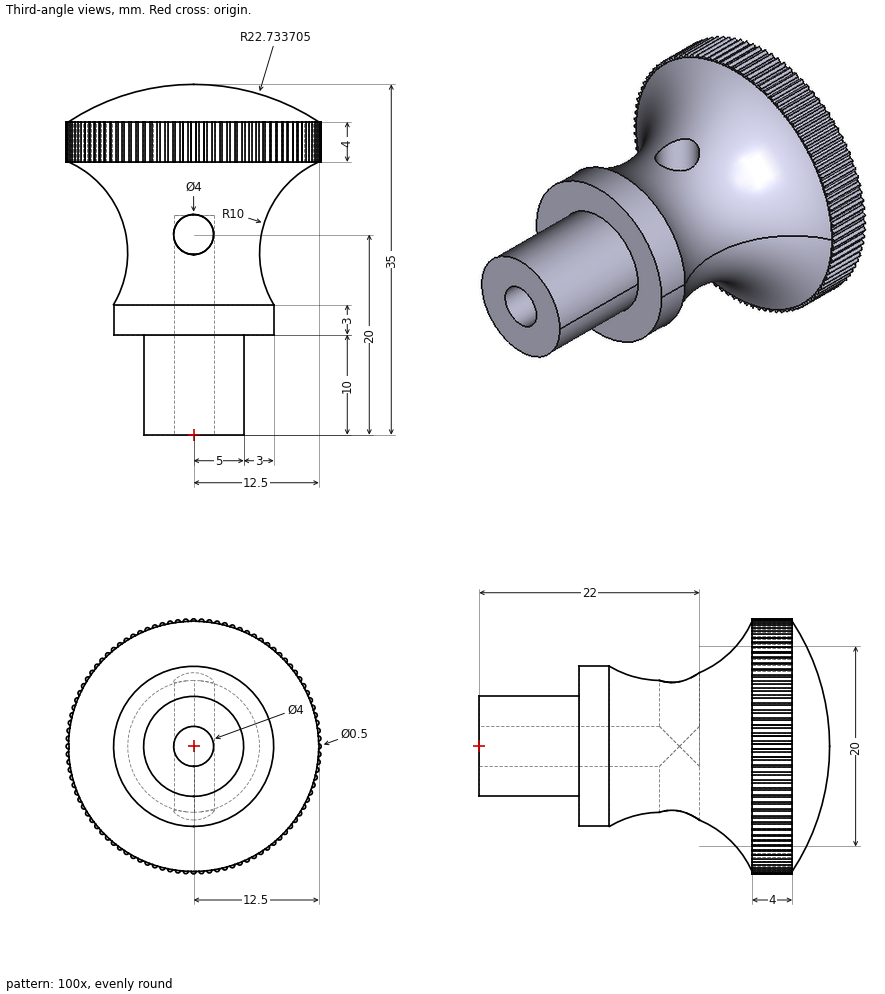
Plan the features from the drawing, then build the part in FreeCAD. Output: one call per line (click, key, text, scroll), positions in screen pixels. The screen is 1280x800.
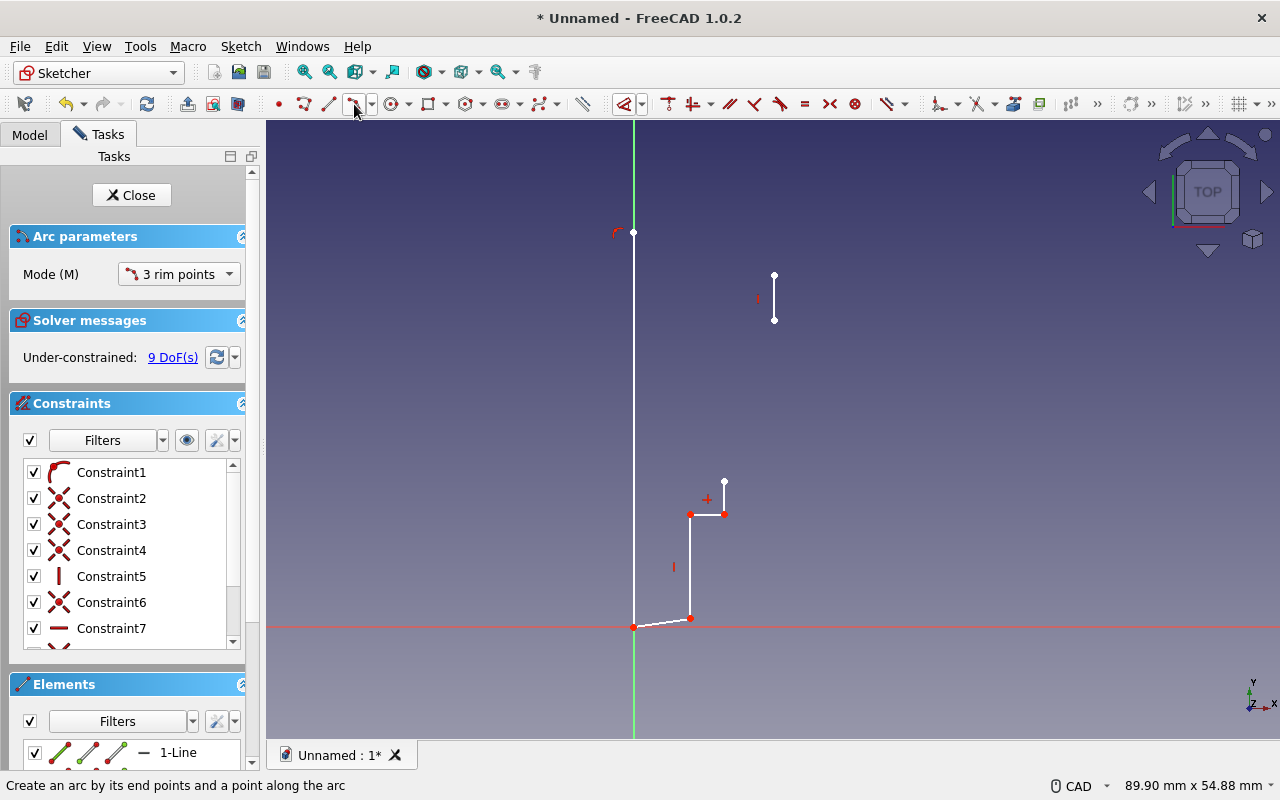
click(724, 482)
click(774, 321)
click(713, 389)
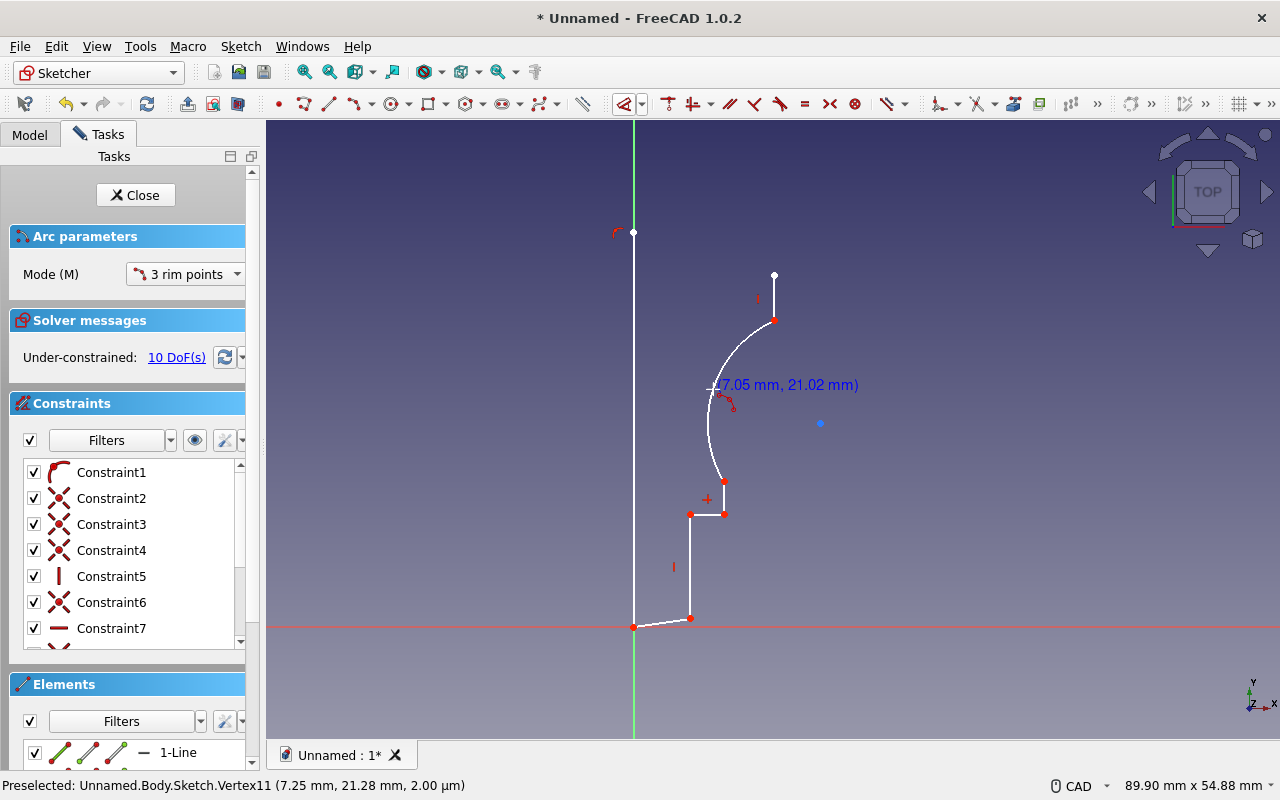
click(774, 276)
click(634, 233)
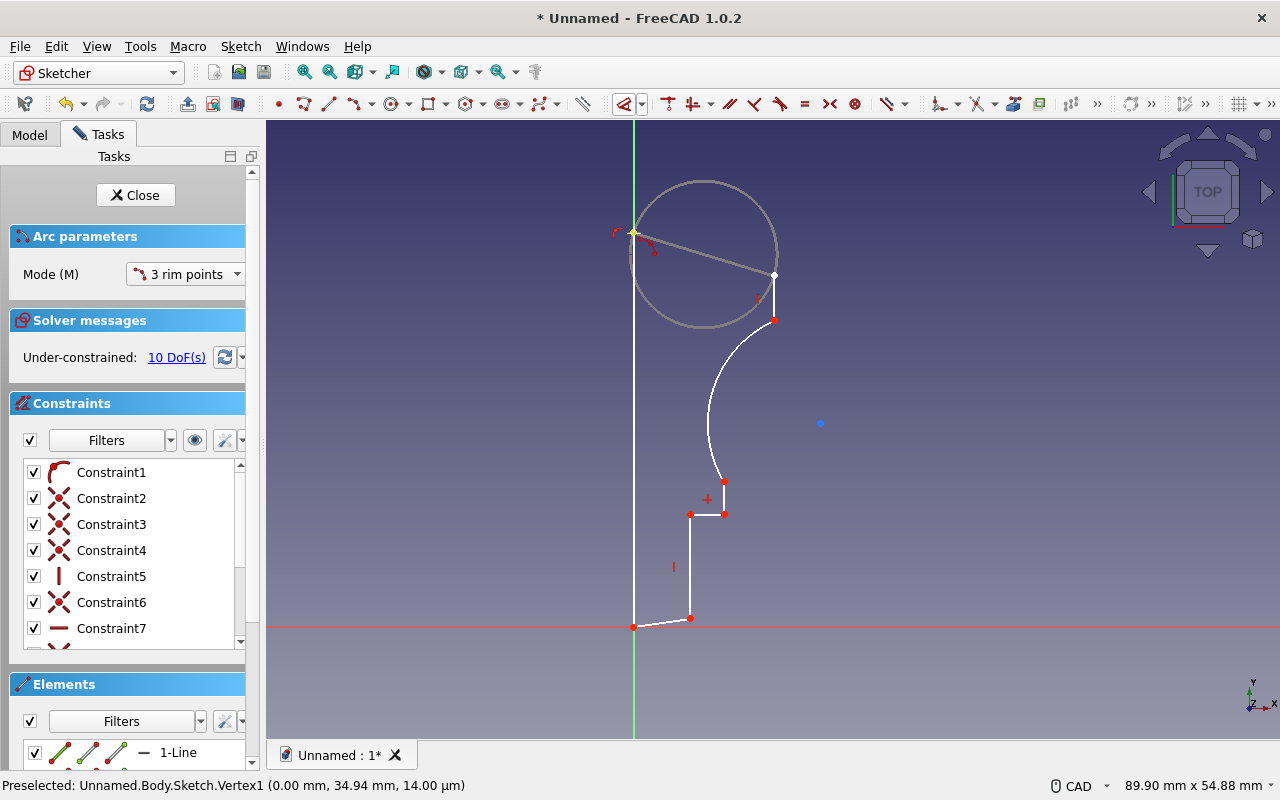
scroll(707, 243, up, 2)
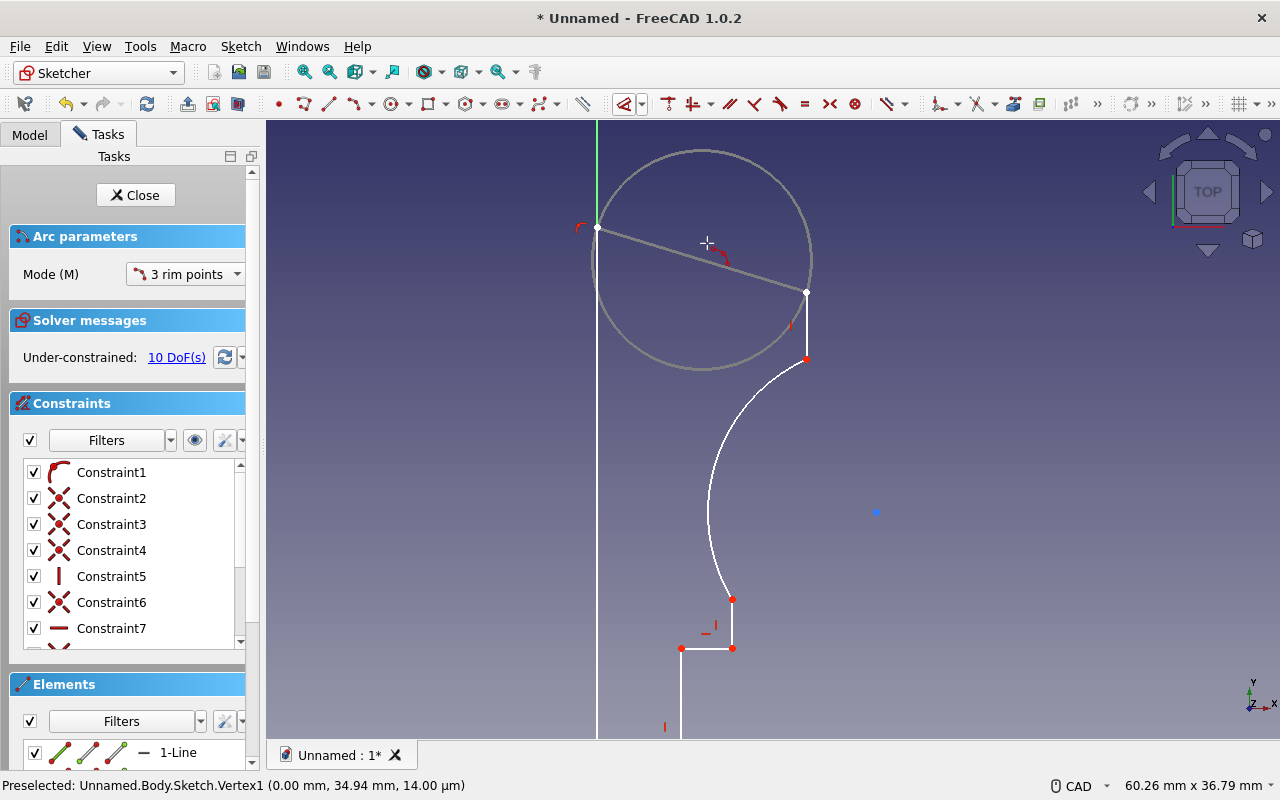
click(707, 243)
key(Escape)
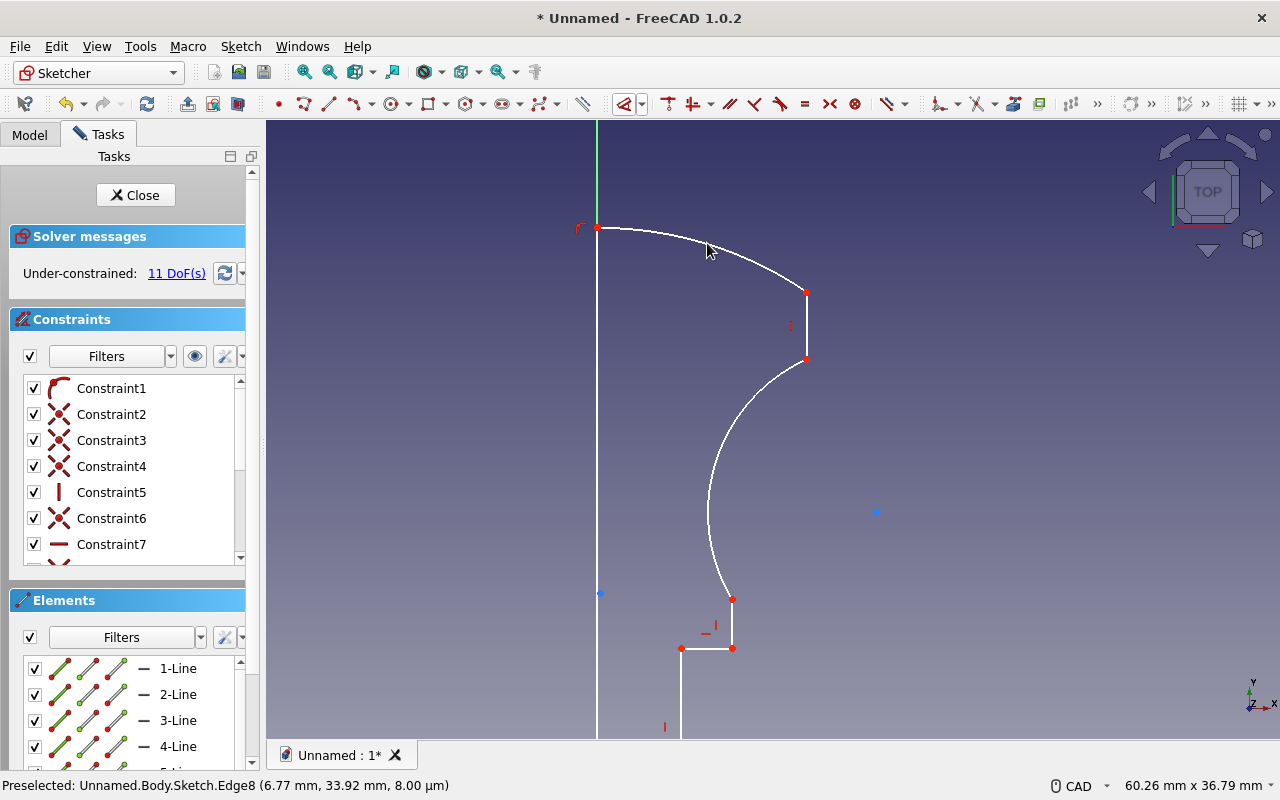
scroll(709, 242, down, 2)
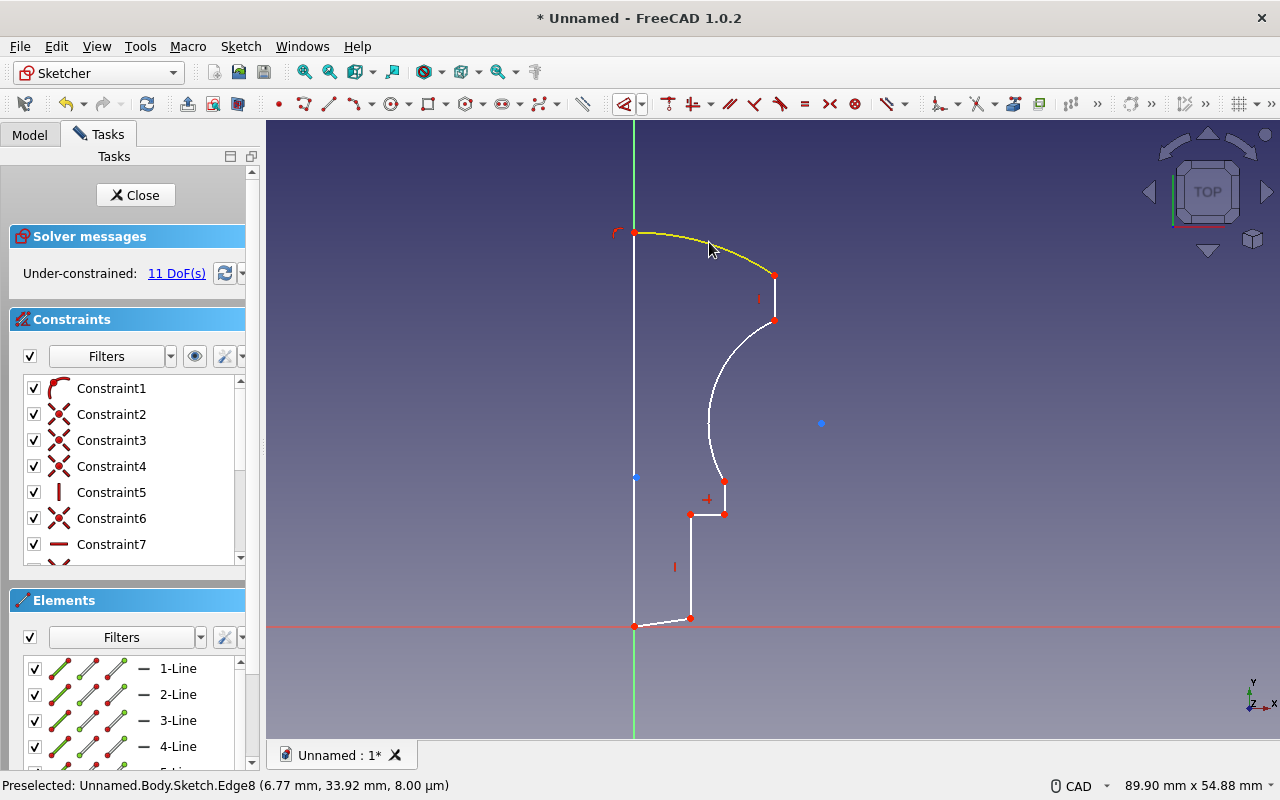
click(651, 624)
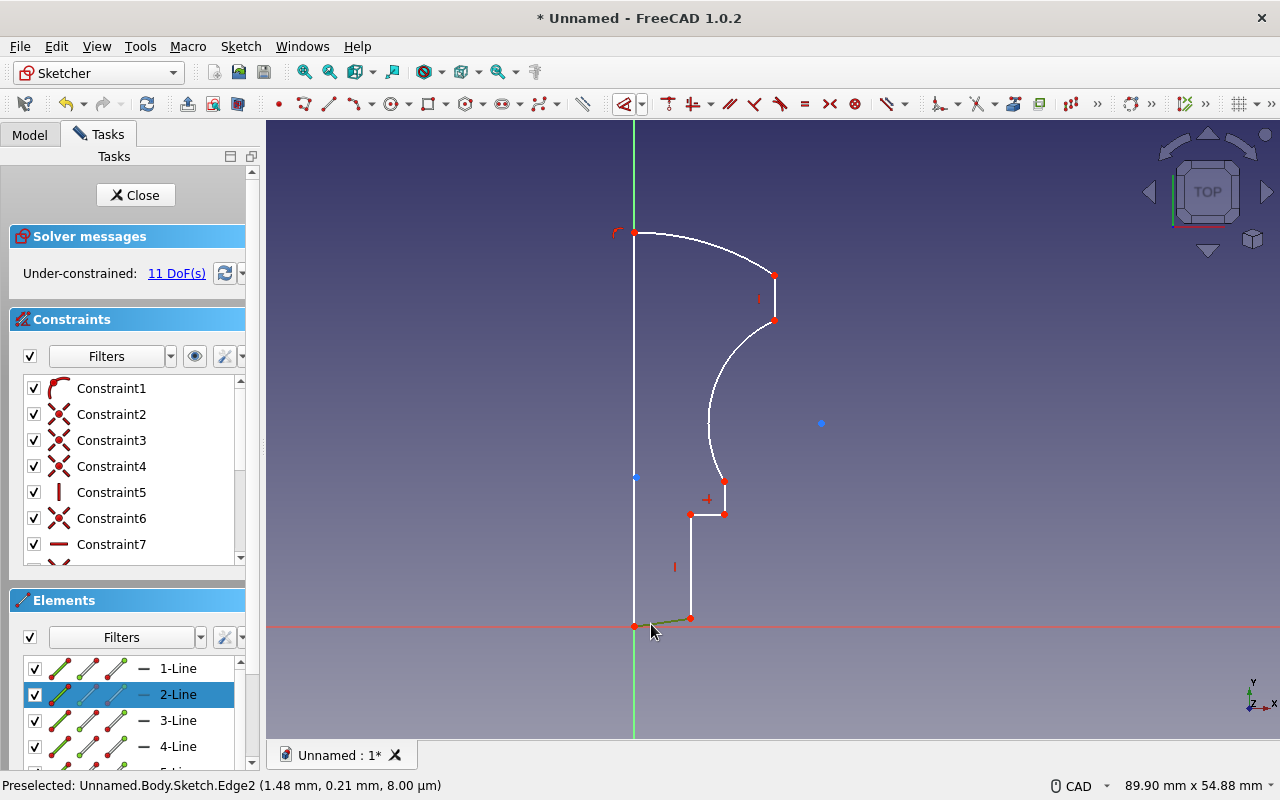
key(h)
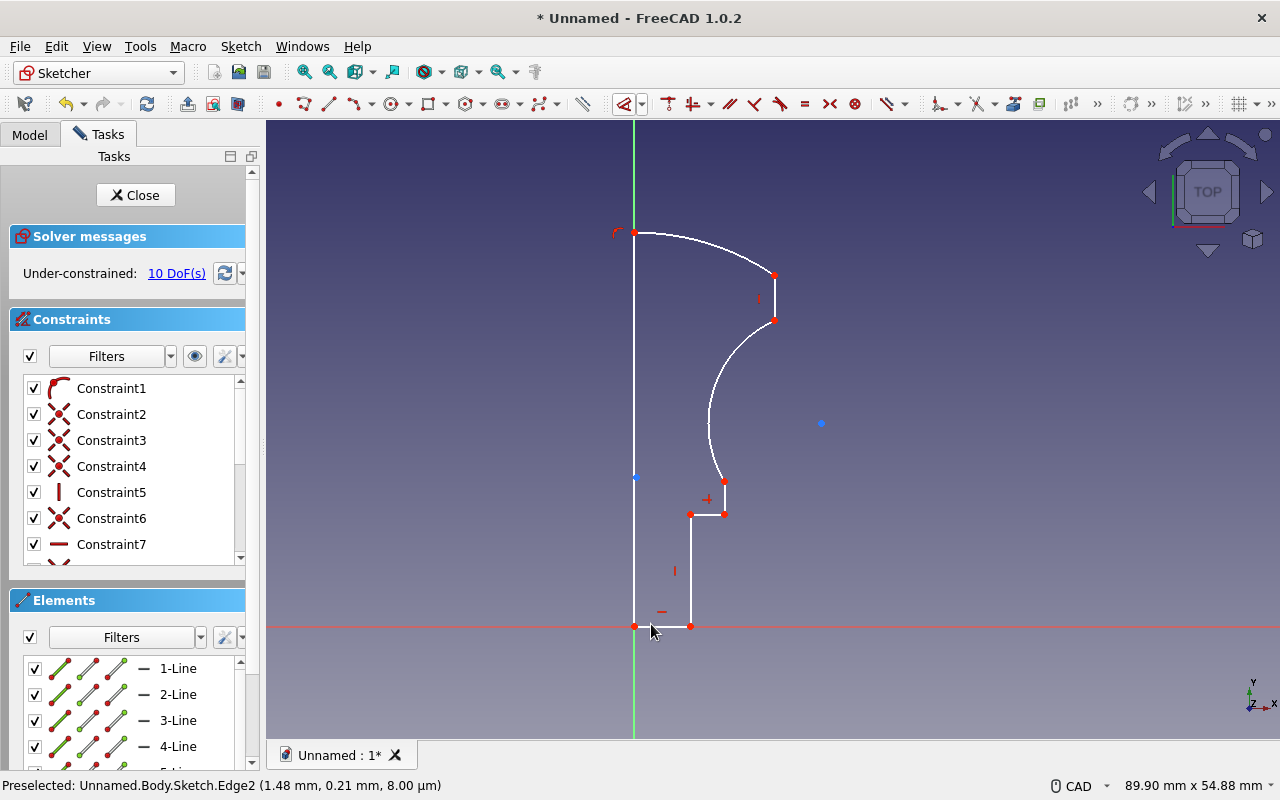
click(636, 477)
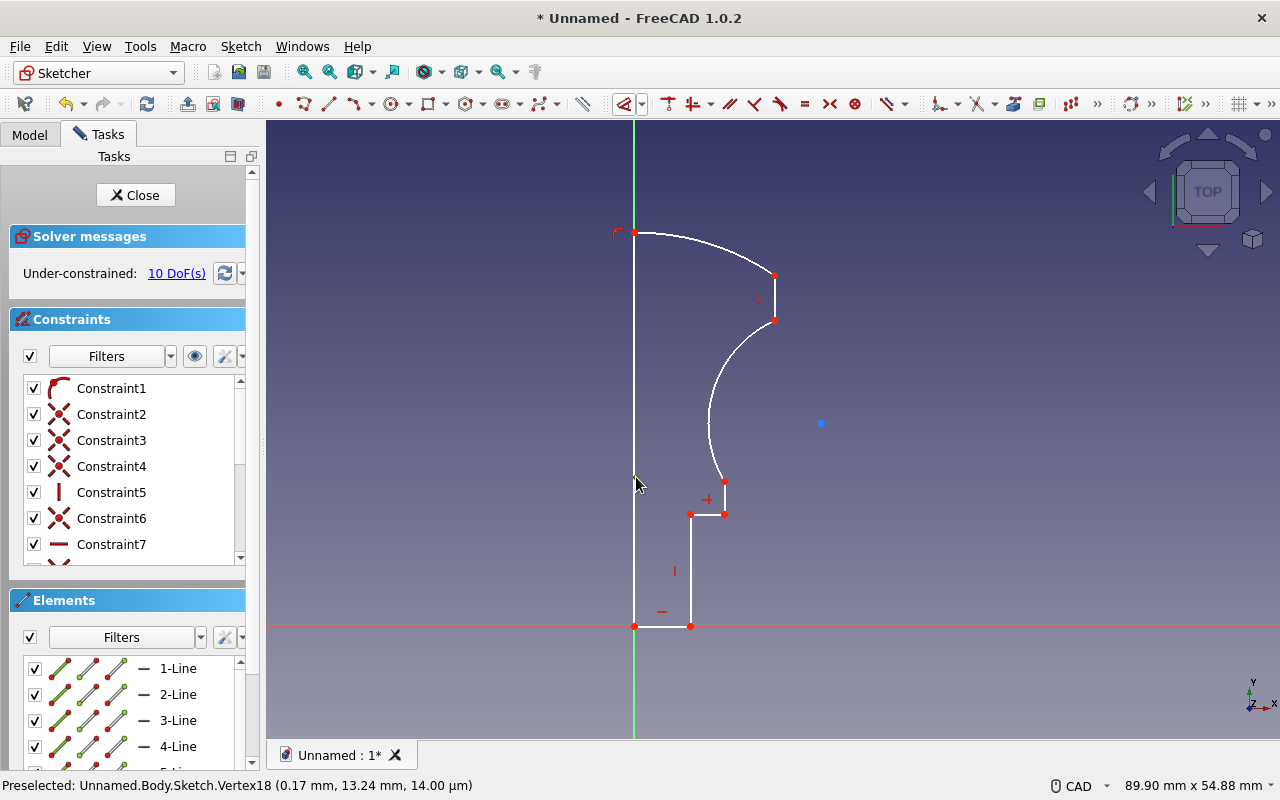
click(634, 671)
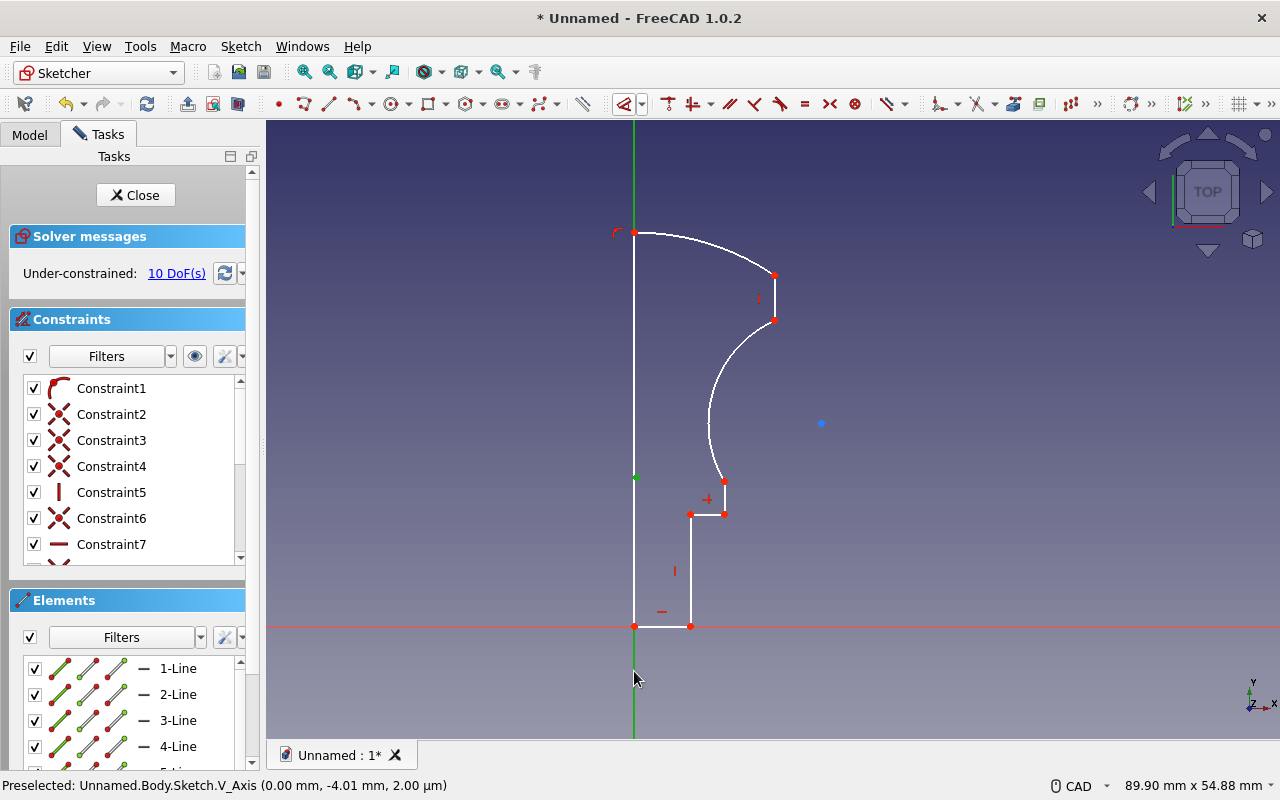
click(668, 104)